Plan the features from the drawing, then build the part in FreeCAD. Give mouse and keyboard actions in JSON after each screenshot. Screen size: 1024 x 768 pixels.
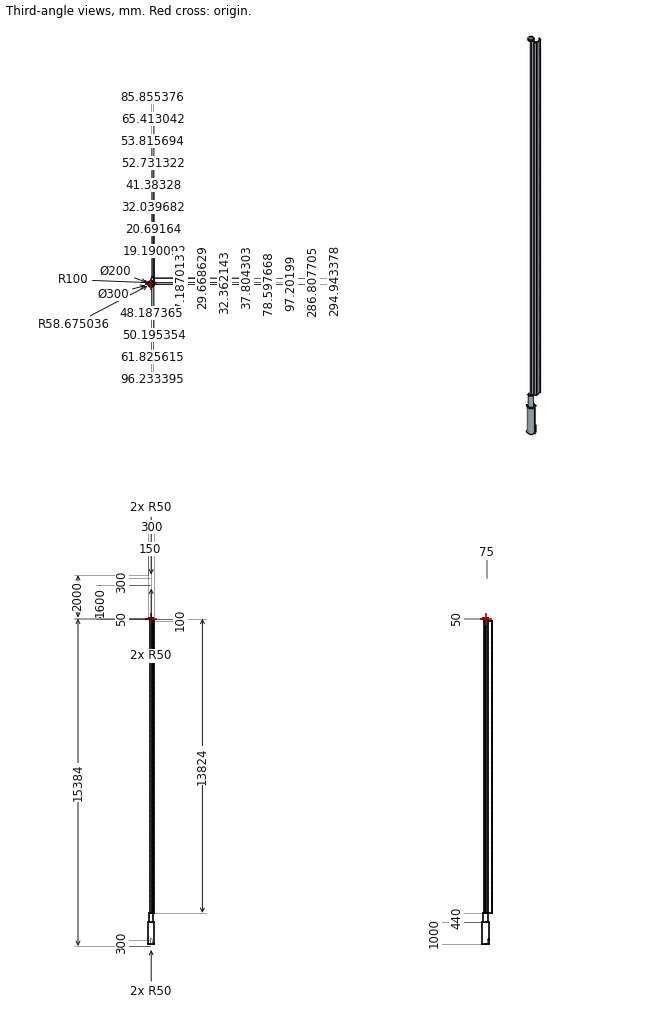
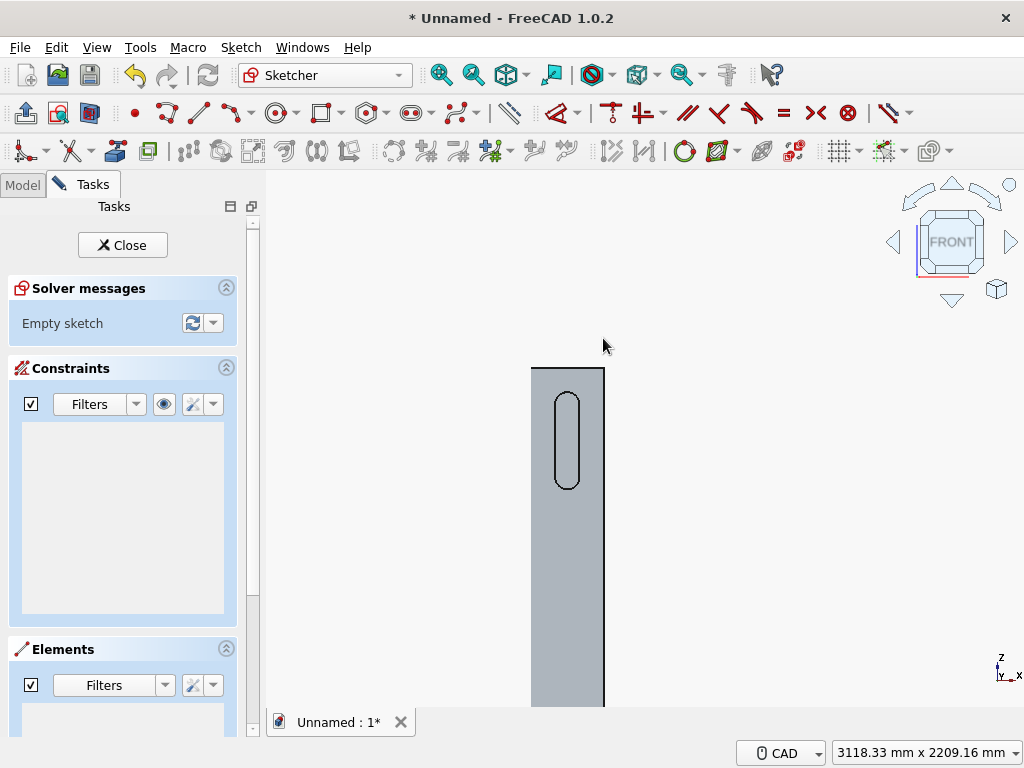
{"action": "scroll", "coordinate": [563, 442], "scroll_direction": "up", "scroll_amount": 6}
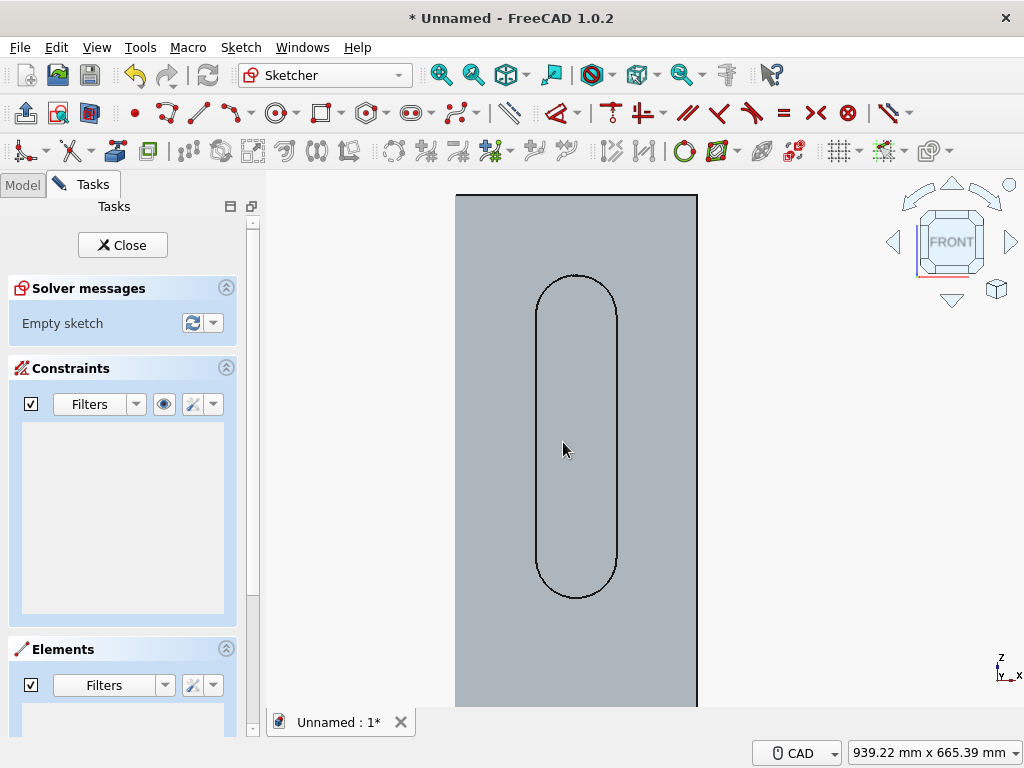
{"action": "left_click", "coordinate": [412, 114]}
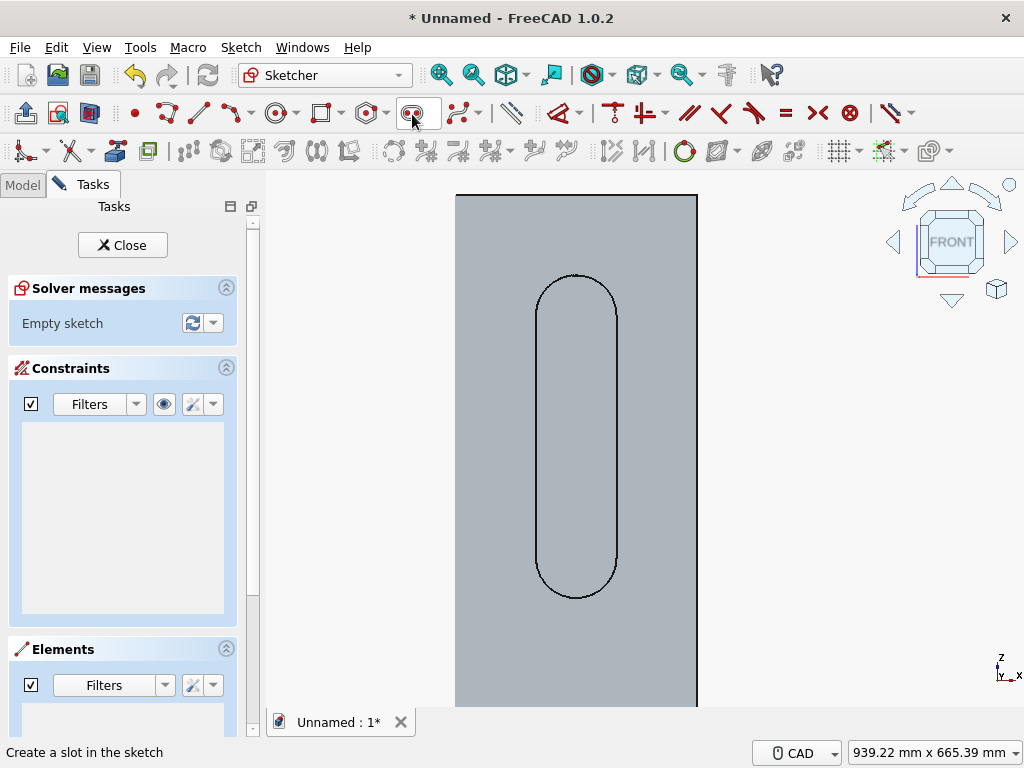
{"action": "left_click", "coordinate": [576, 558]}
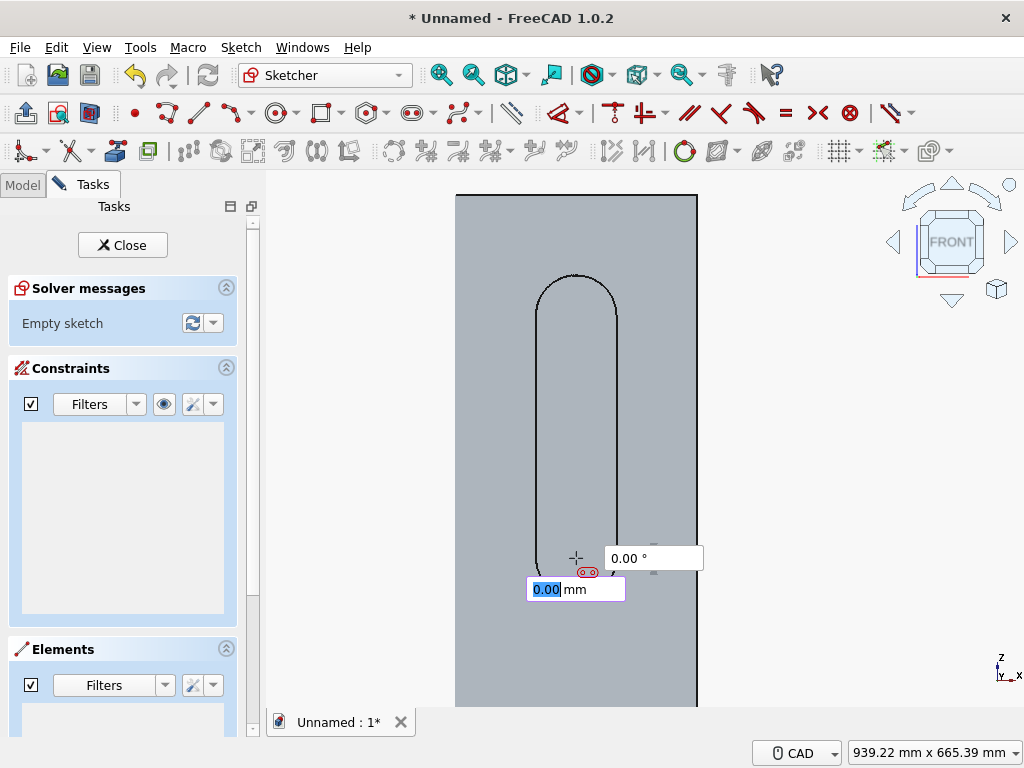
{"action": "left_click", "coordinate": [585, 316]}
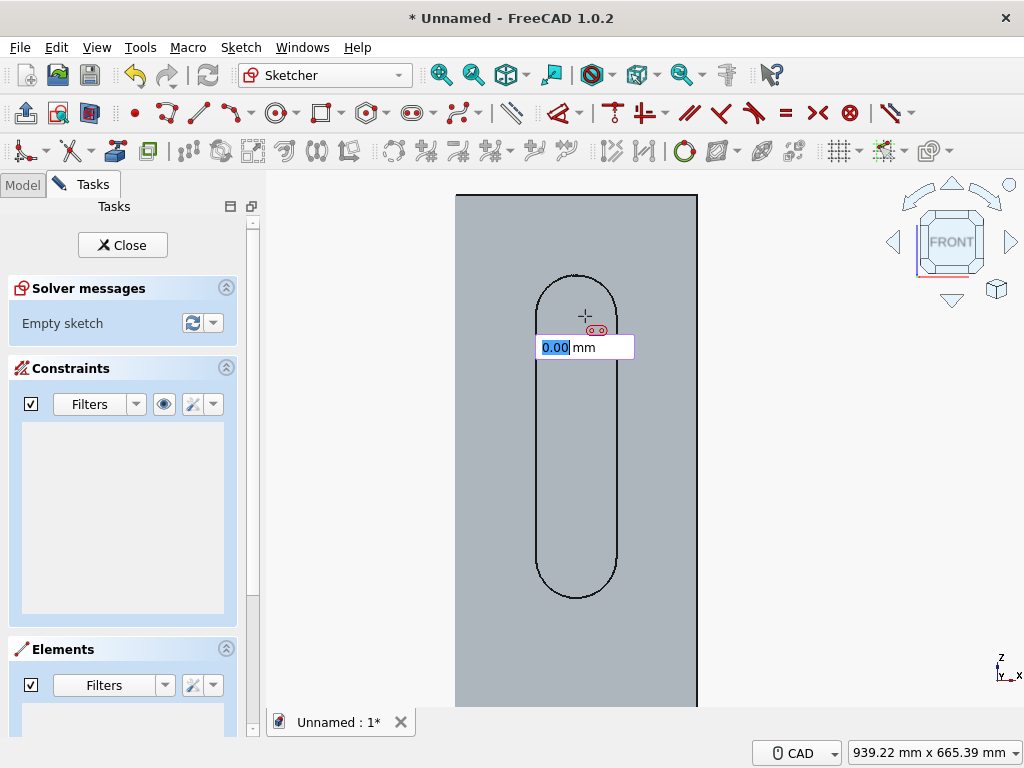
{"action": "left_click", "coordinate": [536, 437]}
{"action": "key", "text": "Escape"}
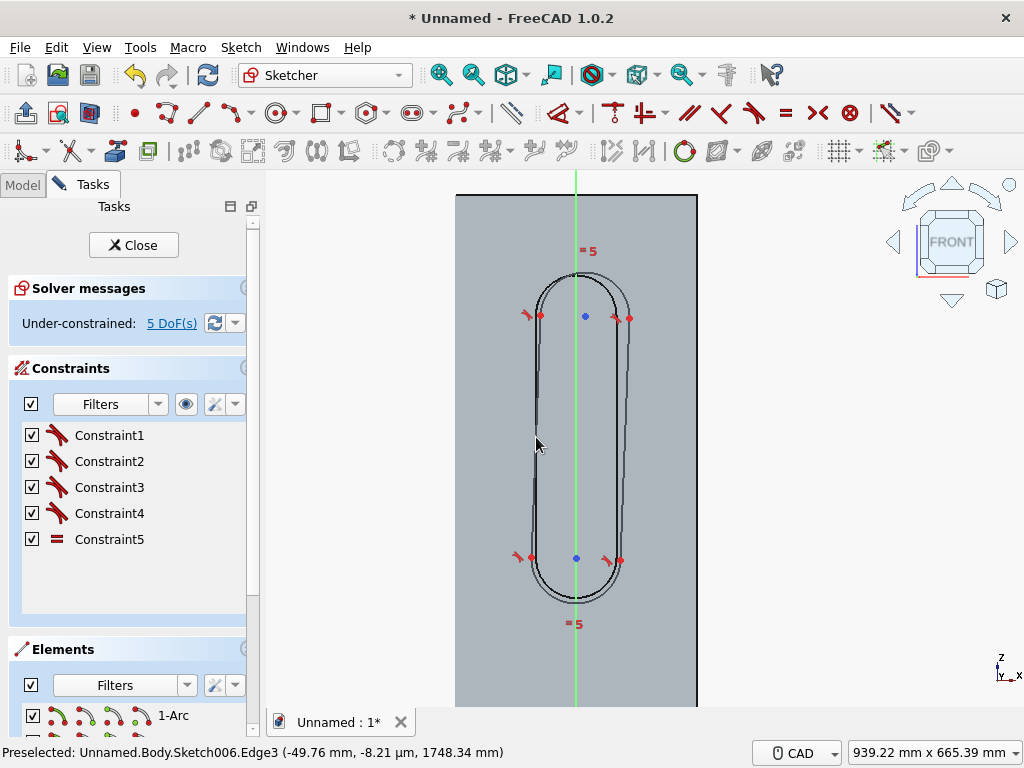
{"action": "left_click", "coordinate": [534, 485]}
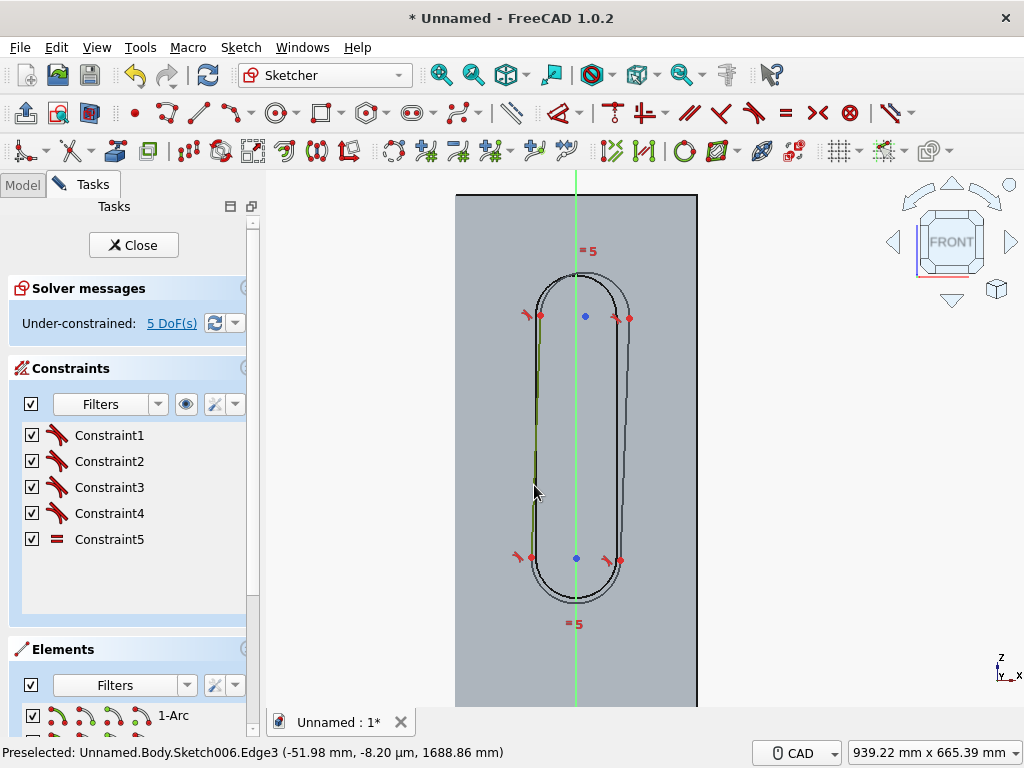
{"action": "key", "text": "v"}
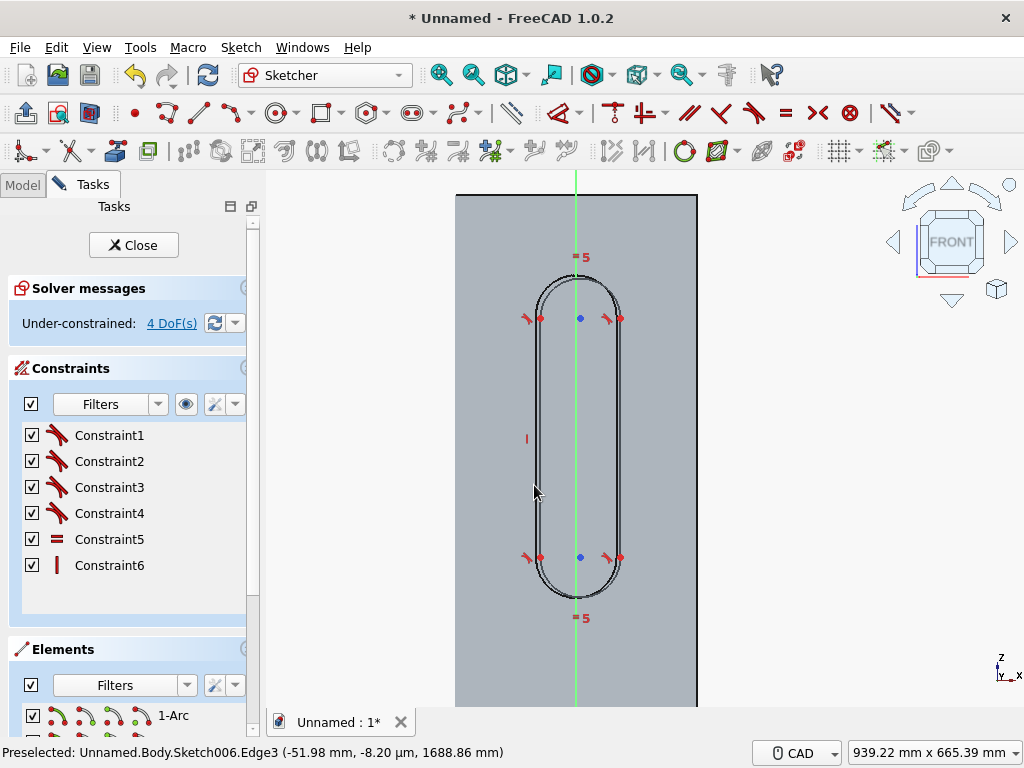
{"action": "left_click", "coordinate": [580, 557]}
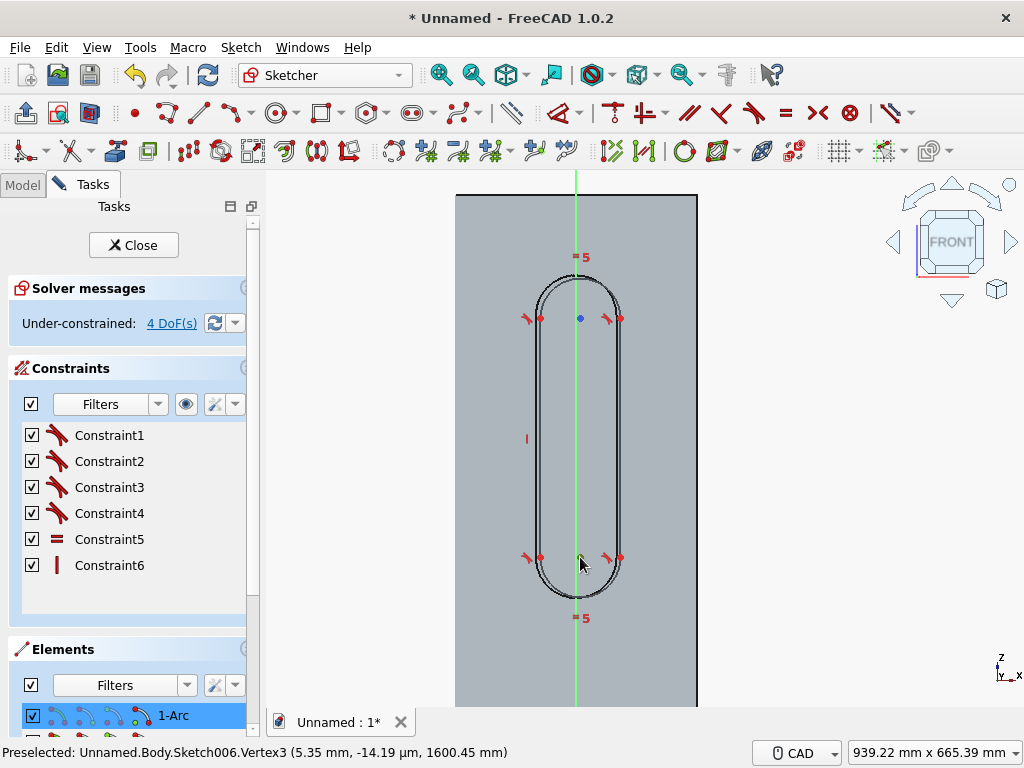
{"action": "left_click", "coordinate": [576, 645]}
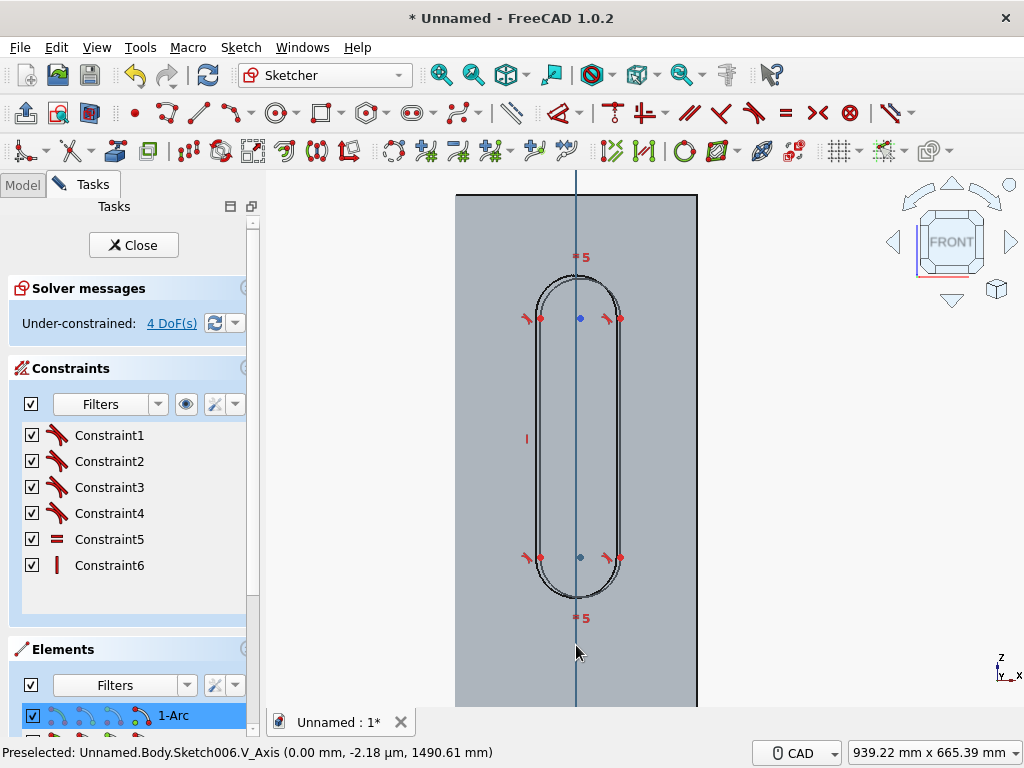
{"action": "left_click", "coordinate": [614, 114]}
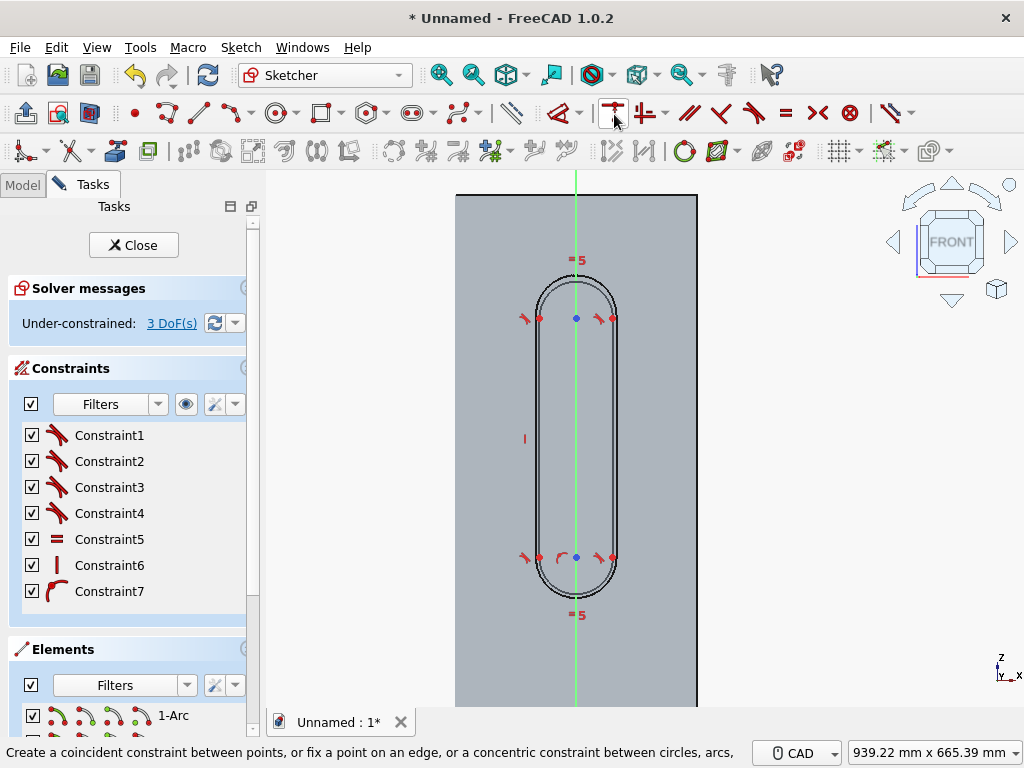
{"action": "left_click", "coordinate": [558, 114]}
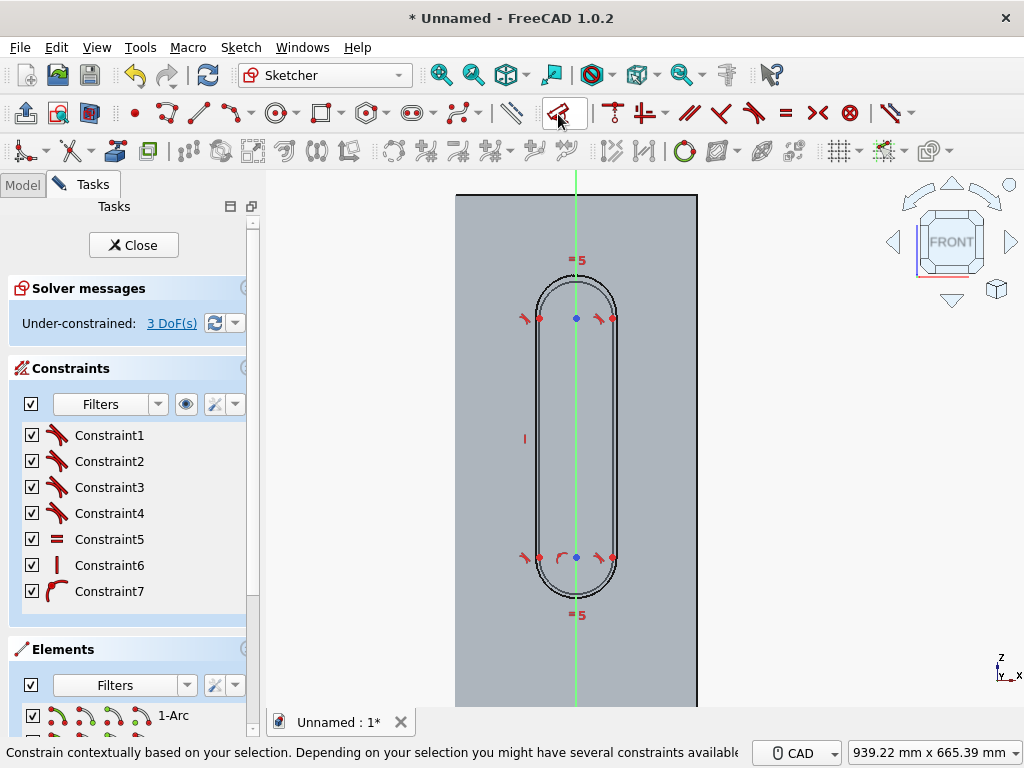
{"action": "left_click", "coordinate": [555, 587]}
{"action": "left_click", "coordinate": [536, 613]}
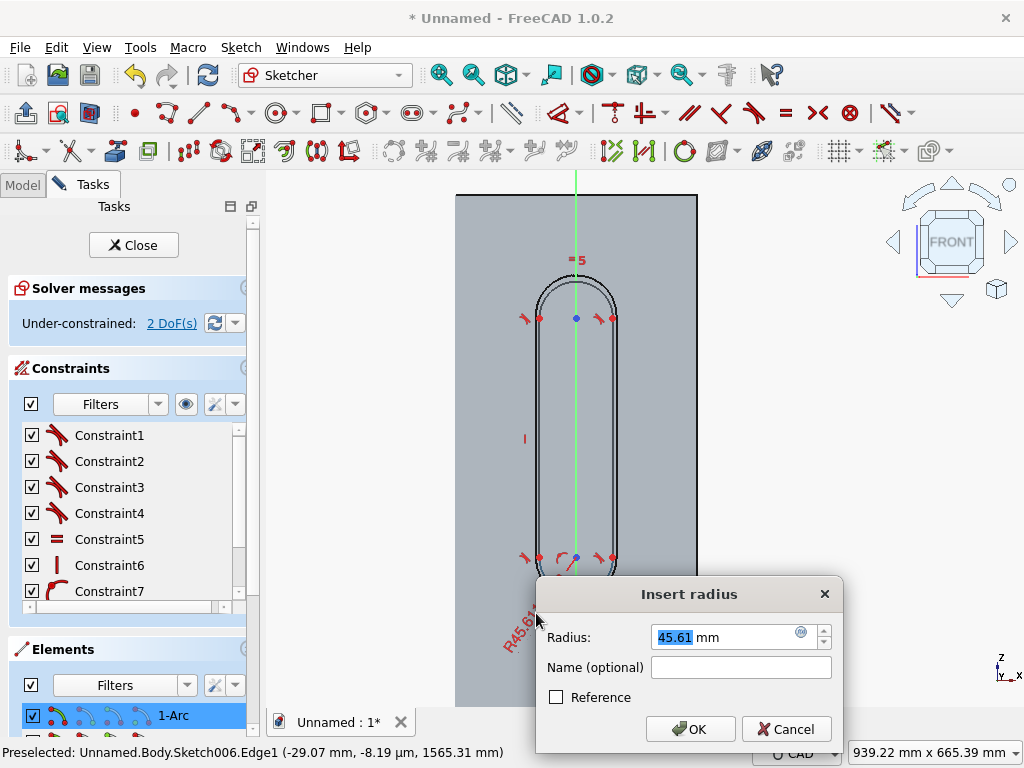
{"action": "type", "text": "50"}
{"action": "key", "text": "Return"}